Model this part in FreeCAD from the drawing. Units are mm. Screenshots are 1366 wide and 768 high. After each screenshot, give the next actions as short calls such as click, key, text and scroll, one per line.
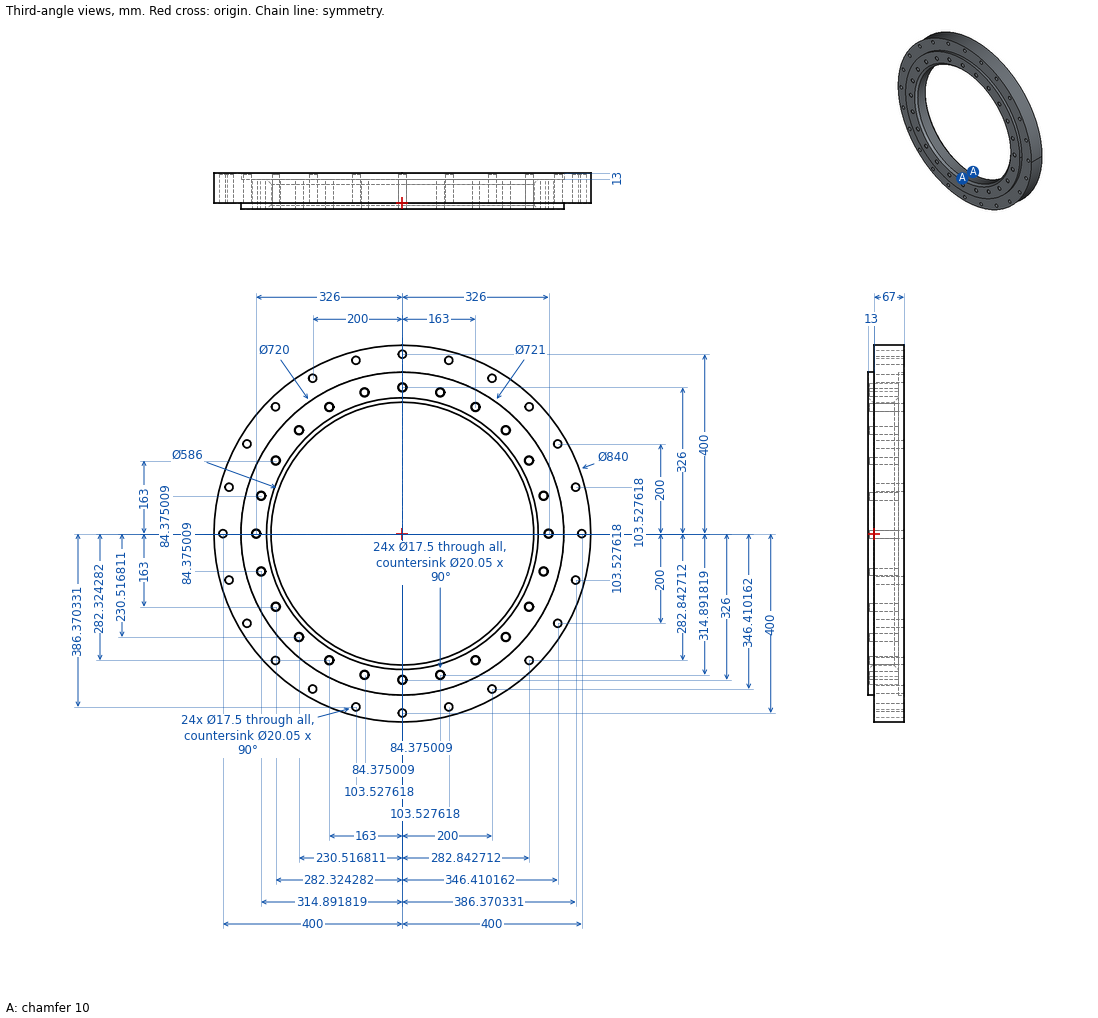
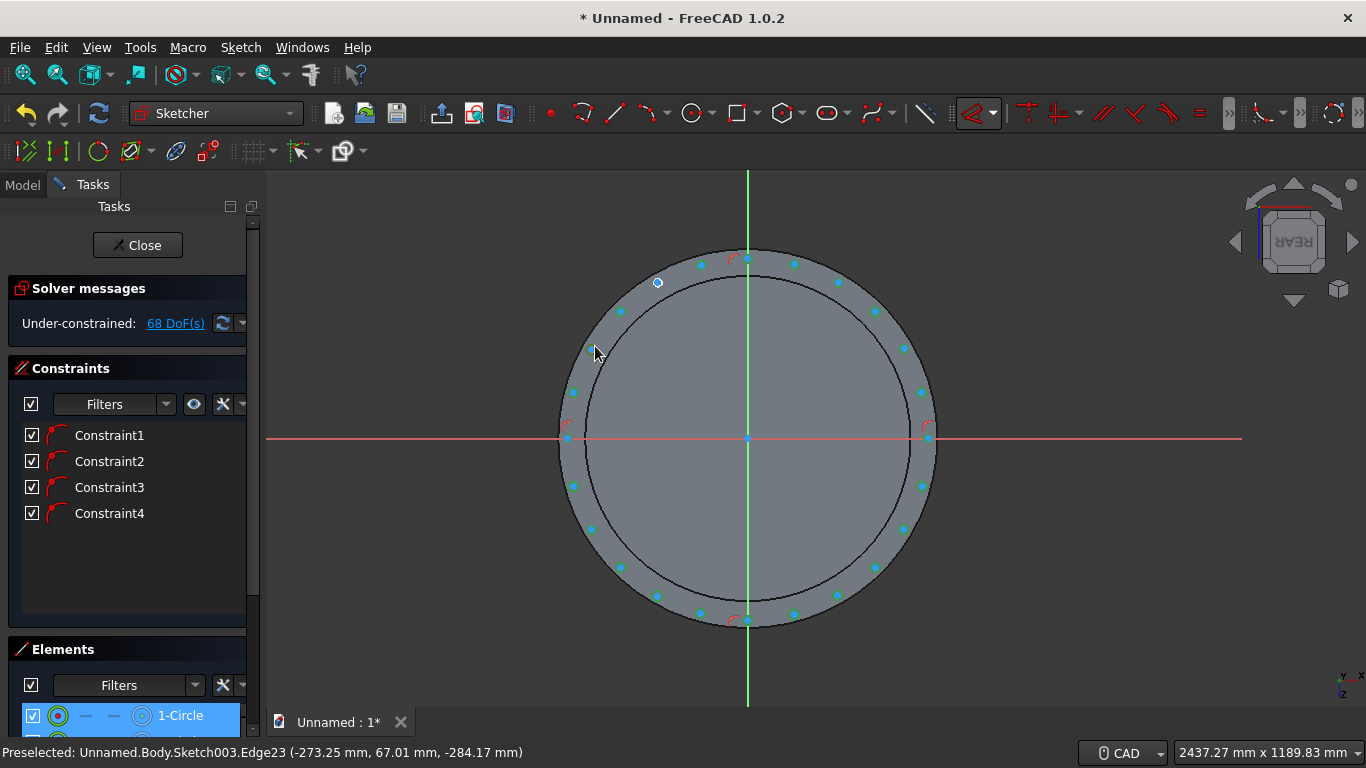
scroll(661, 280, up, 7)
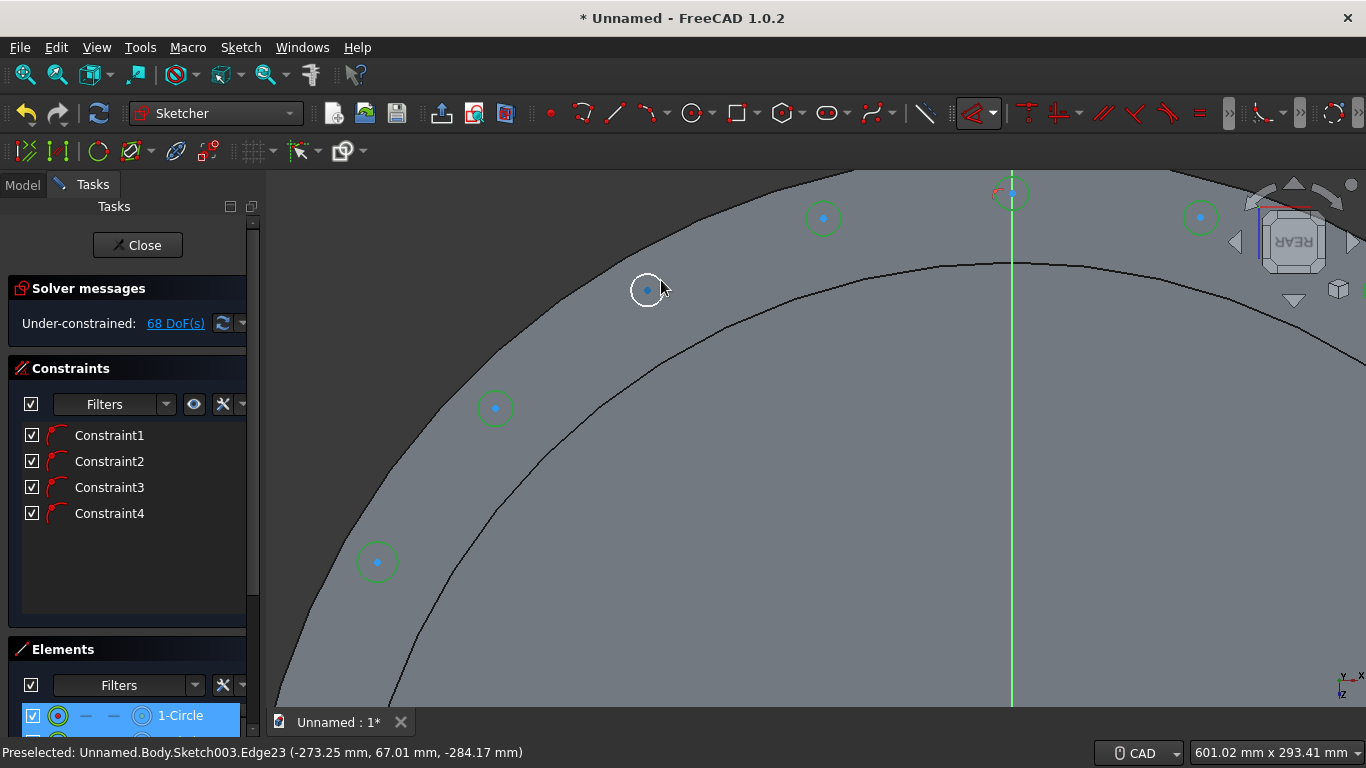
click(659, 279)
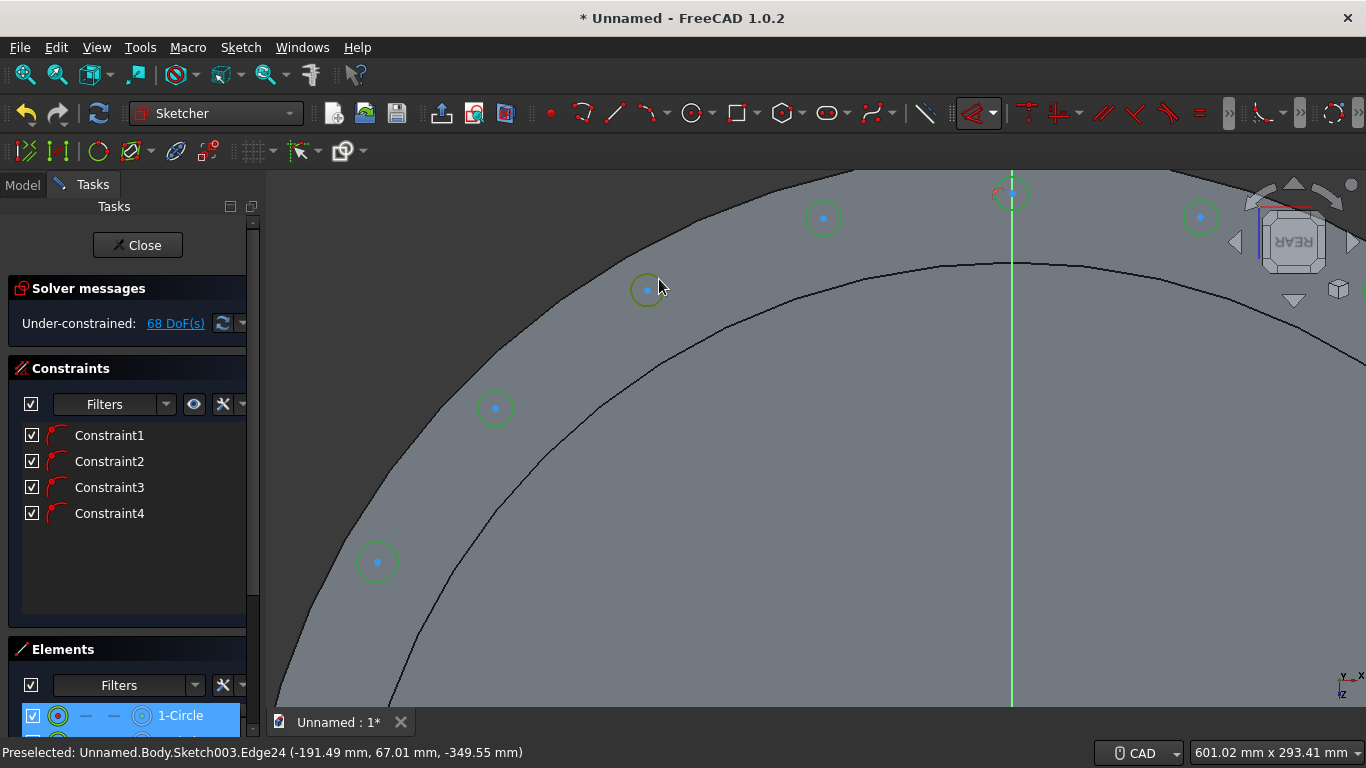
key(e)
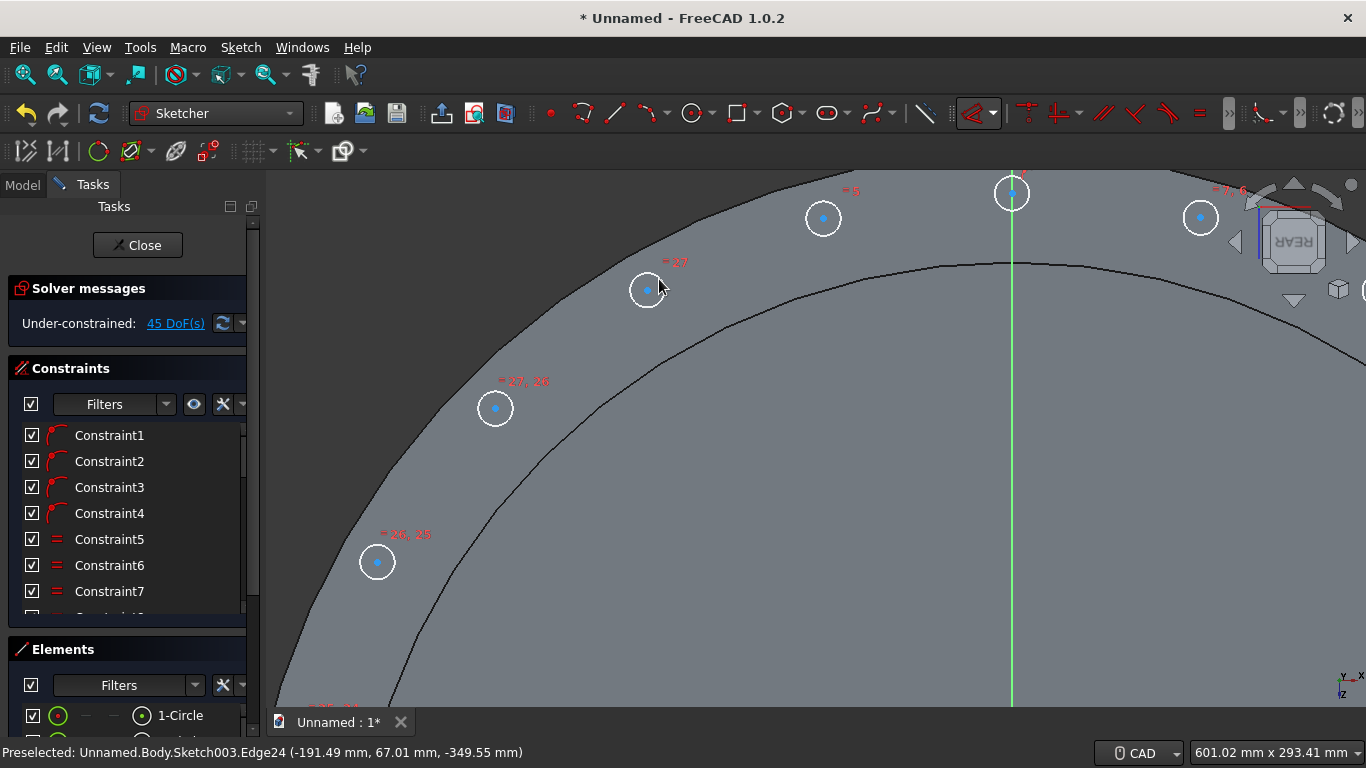
scroll(661, 280, down, 7)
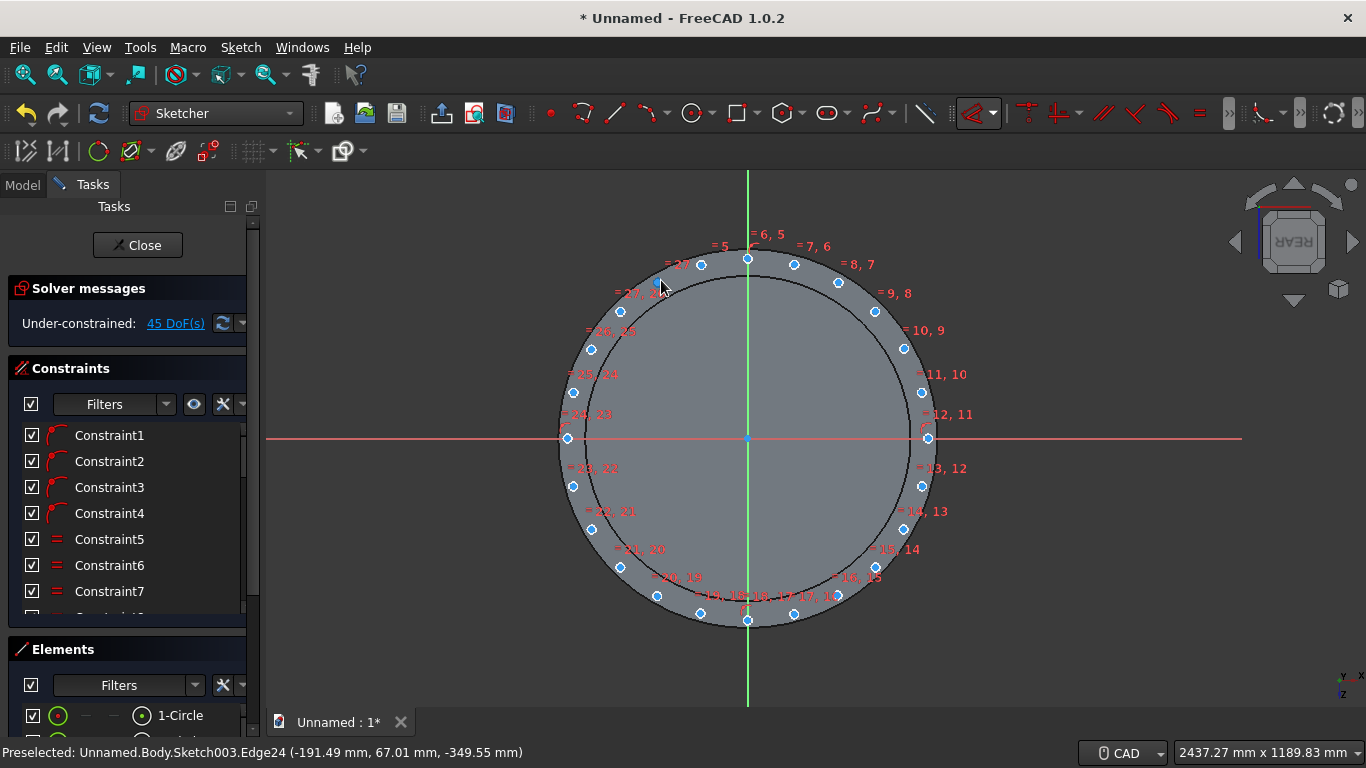
click(701, 265)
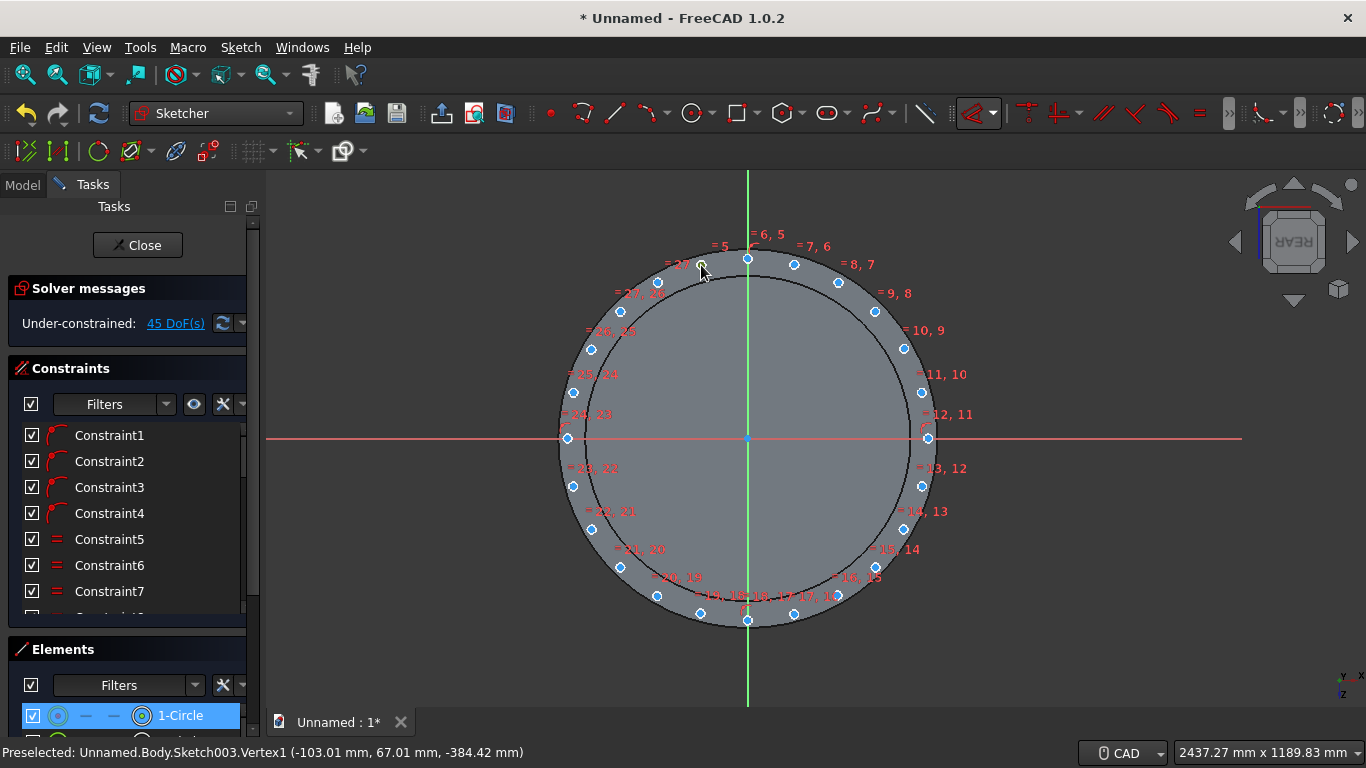
click(794, 265)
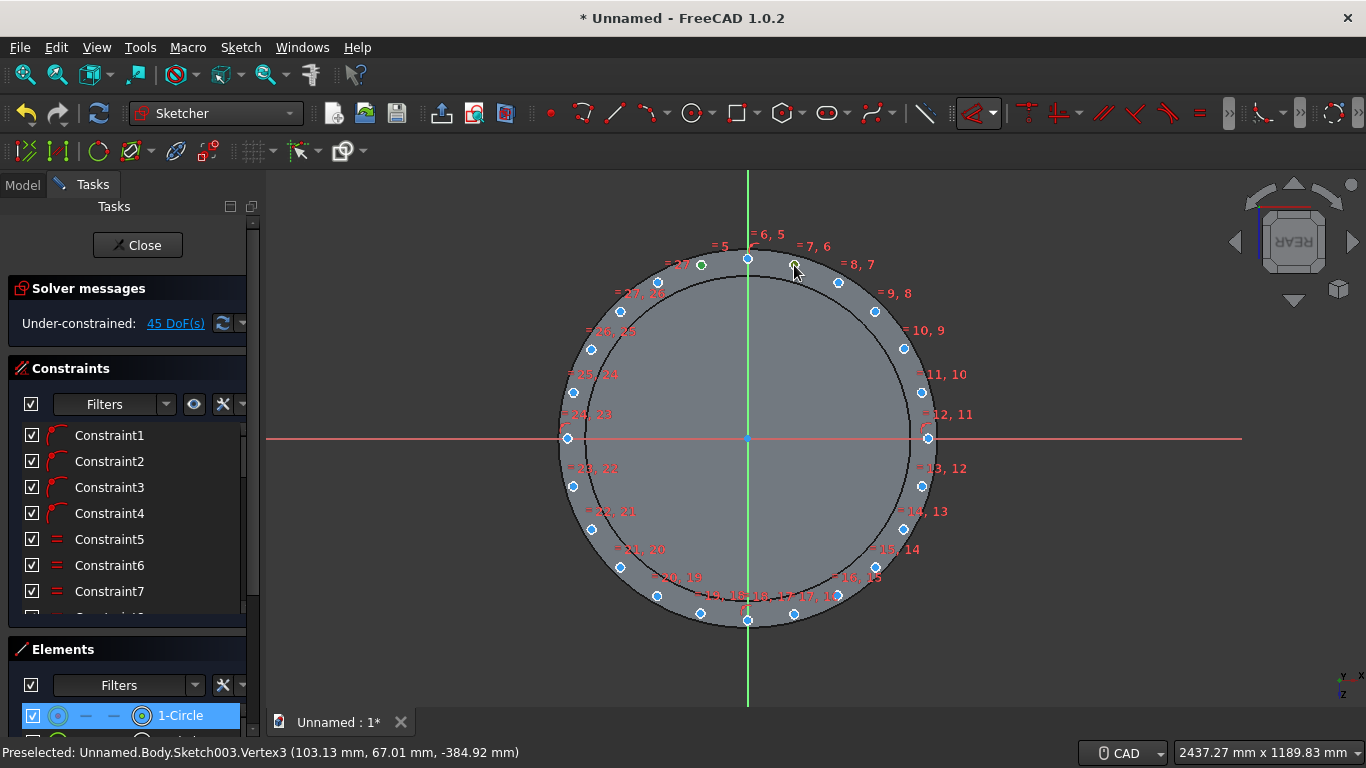
key(h)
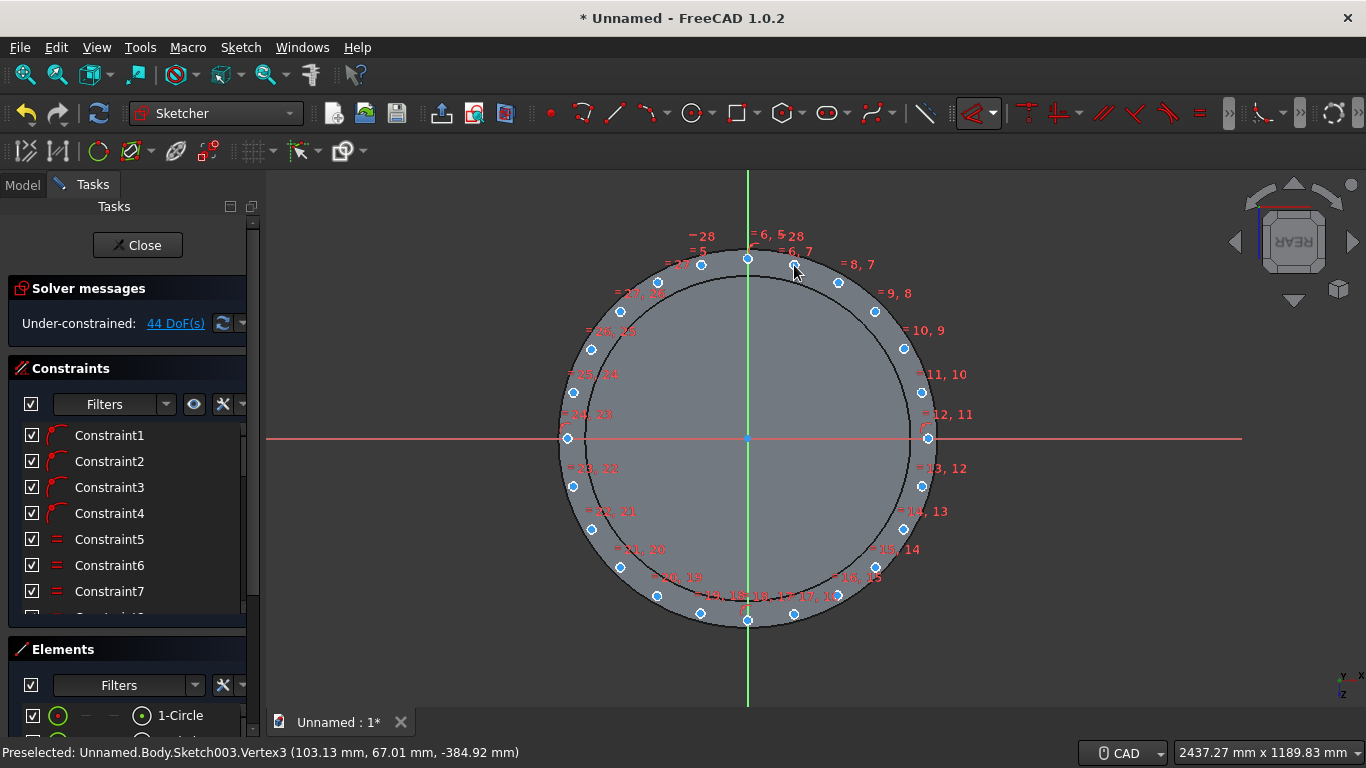
click(922, 393)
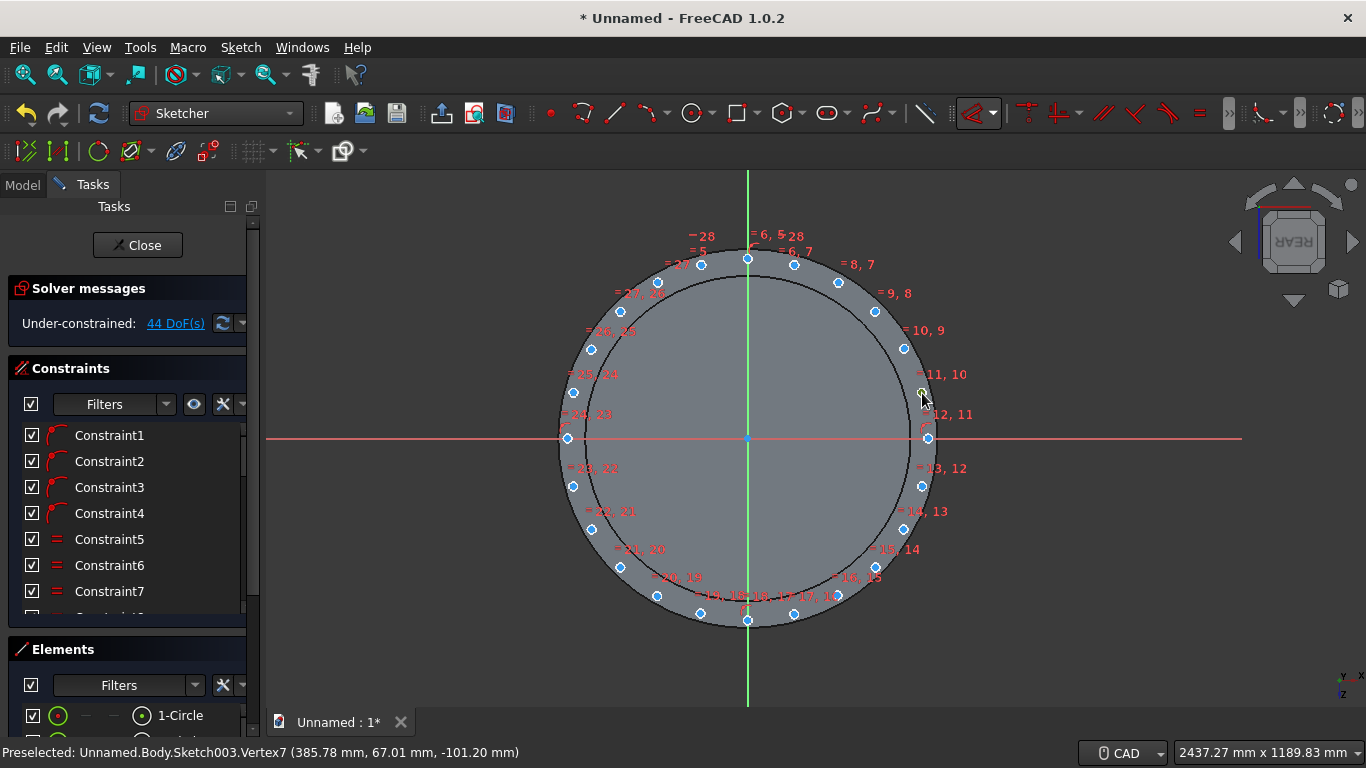
click(922, 486)